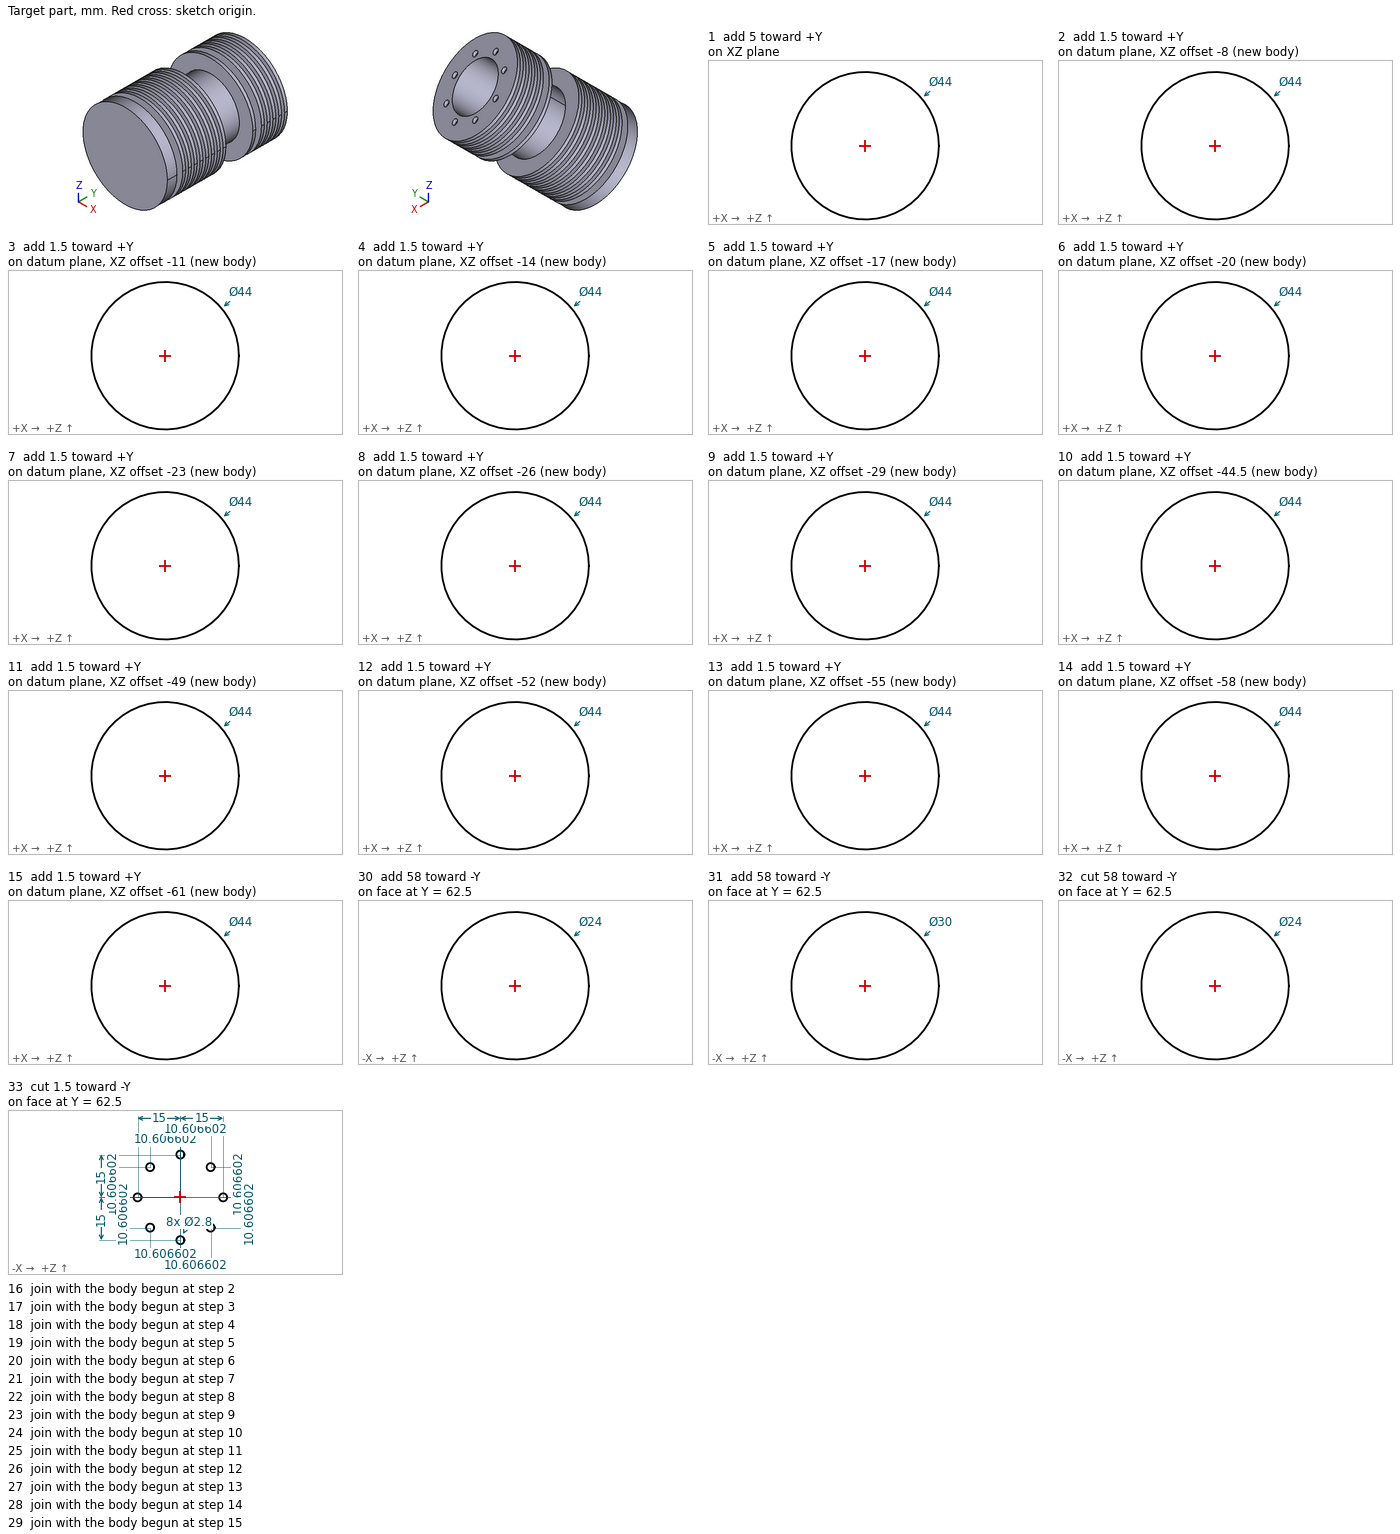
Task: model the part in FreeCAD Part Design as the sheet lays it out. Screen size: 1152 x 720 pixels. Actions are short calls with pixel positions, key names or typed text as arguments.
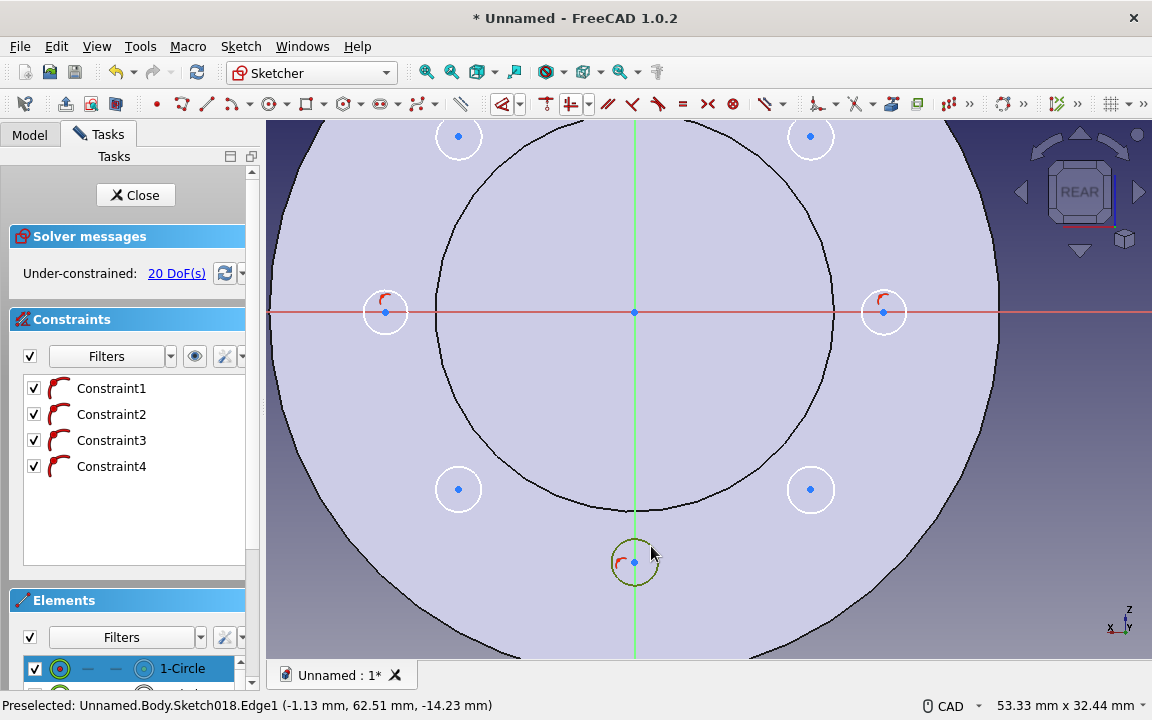
click(475, 473)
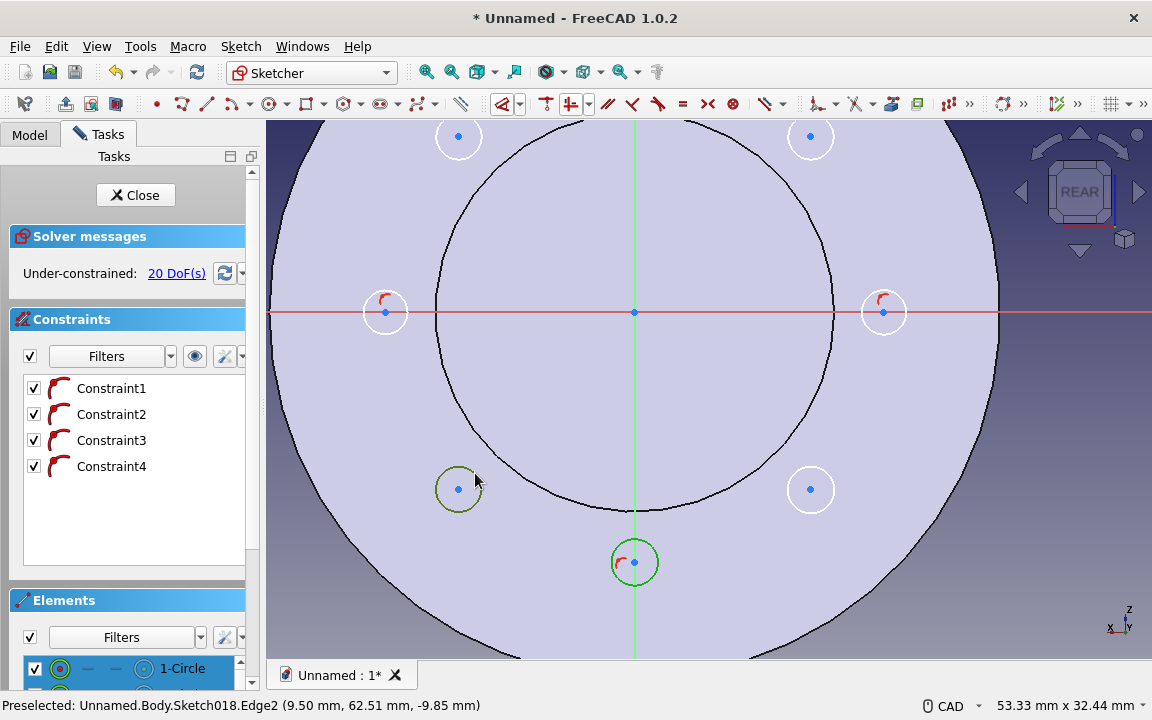
click(401, 297)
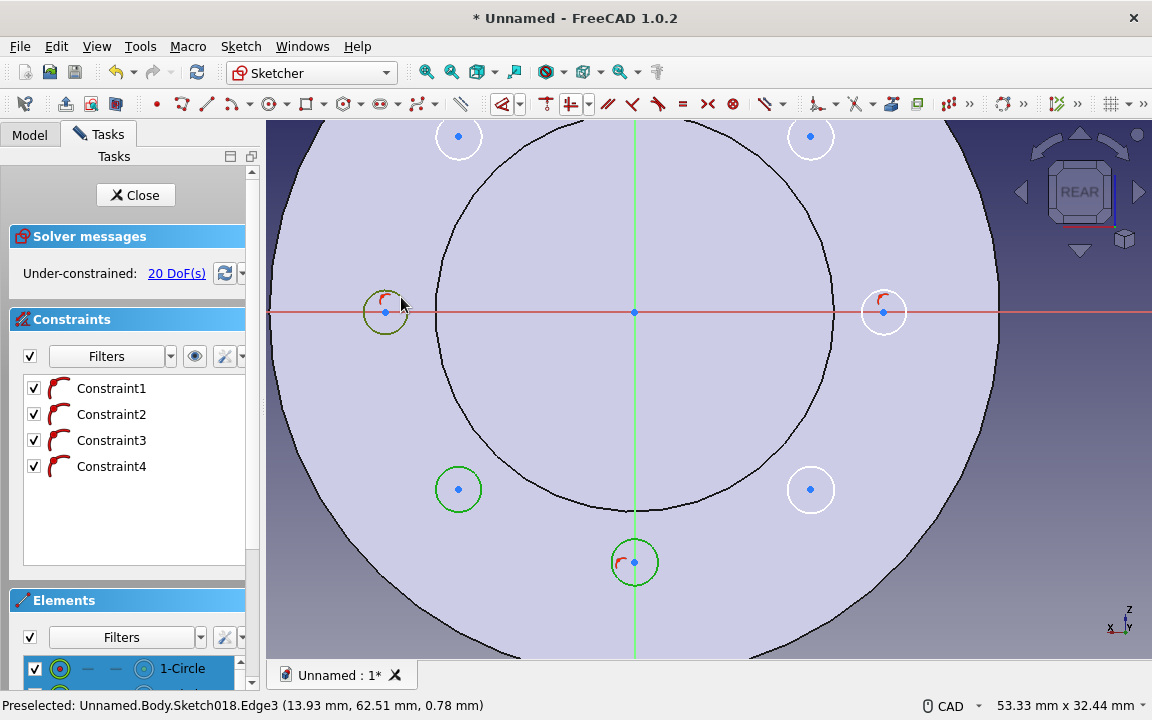
click(443, 153)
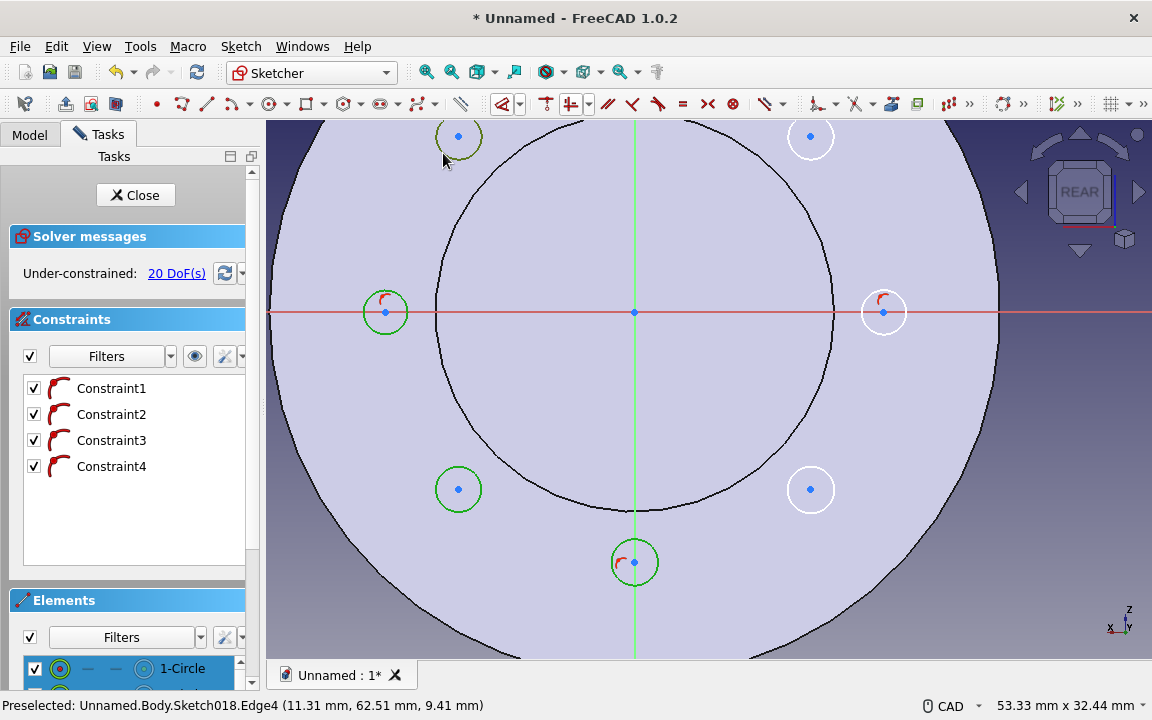
scroll(652, 546, down, 2)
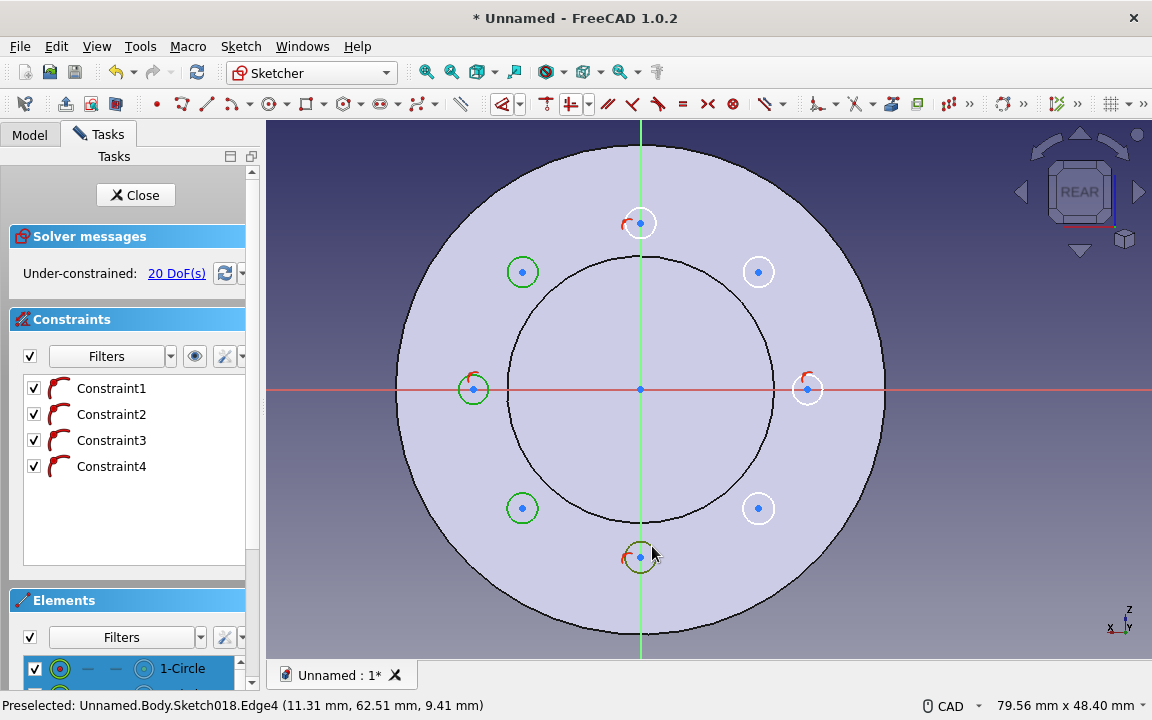
scroll(651, 212, up, 2)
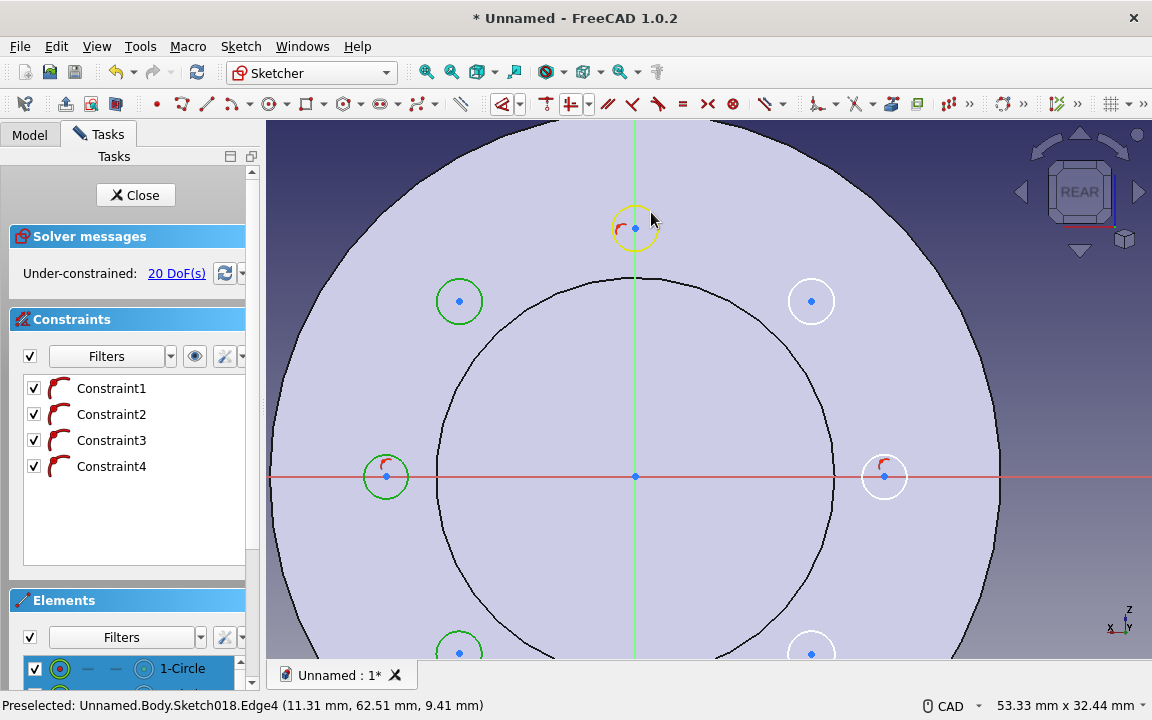
click(651, 212)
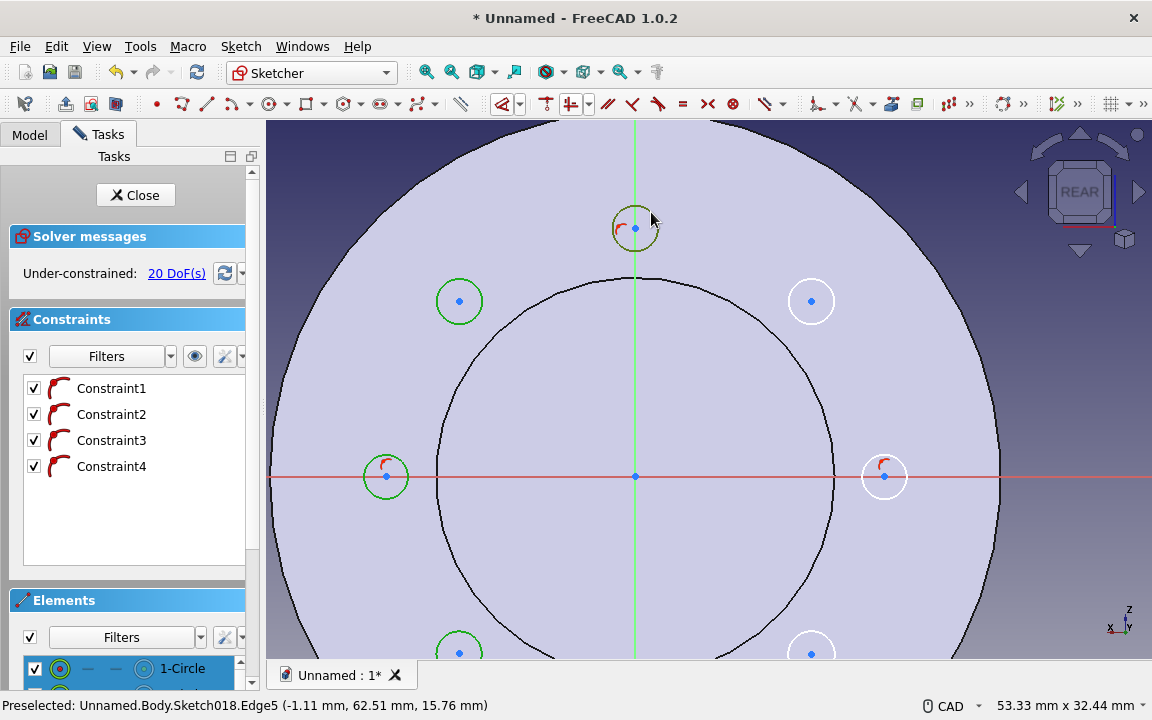
click(827, 286)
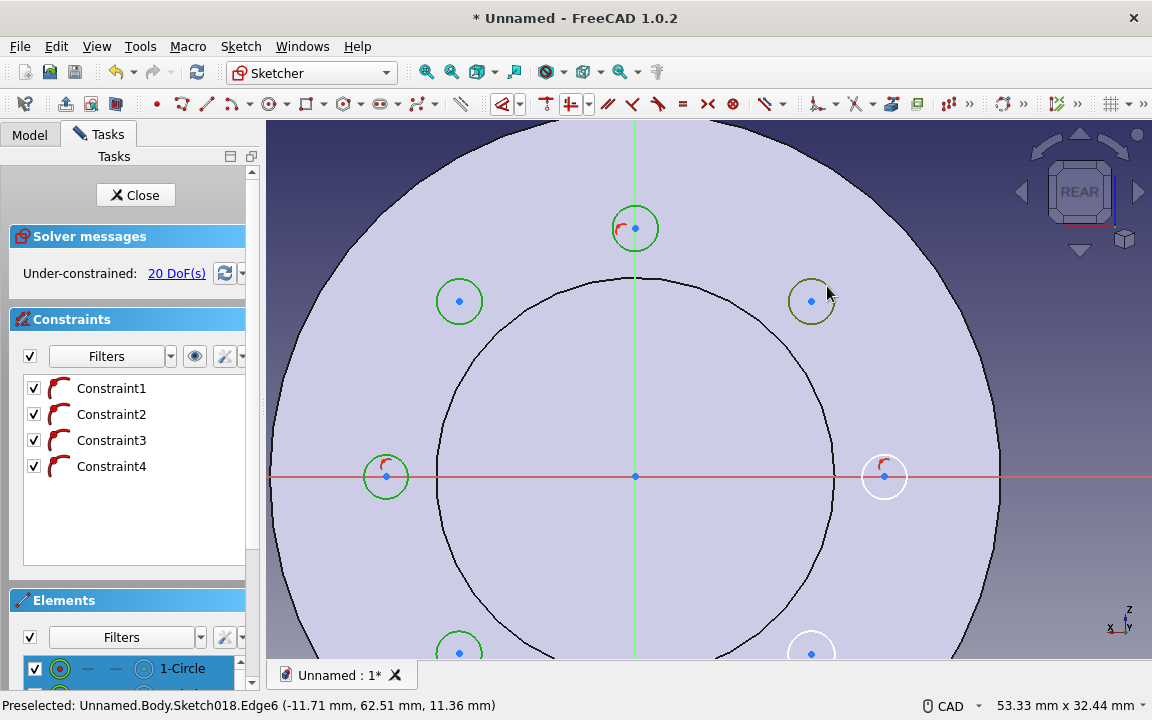
click(900, 461)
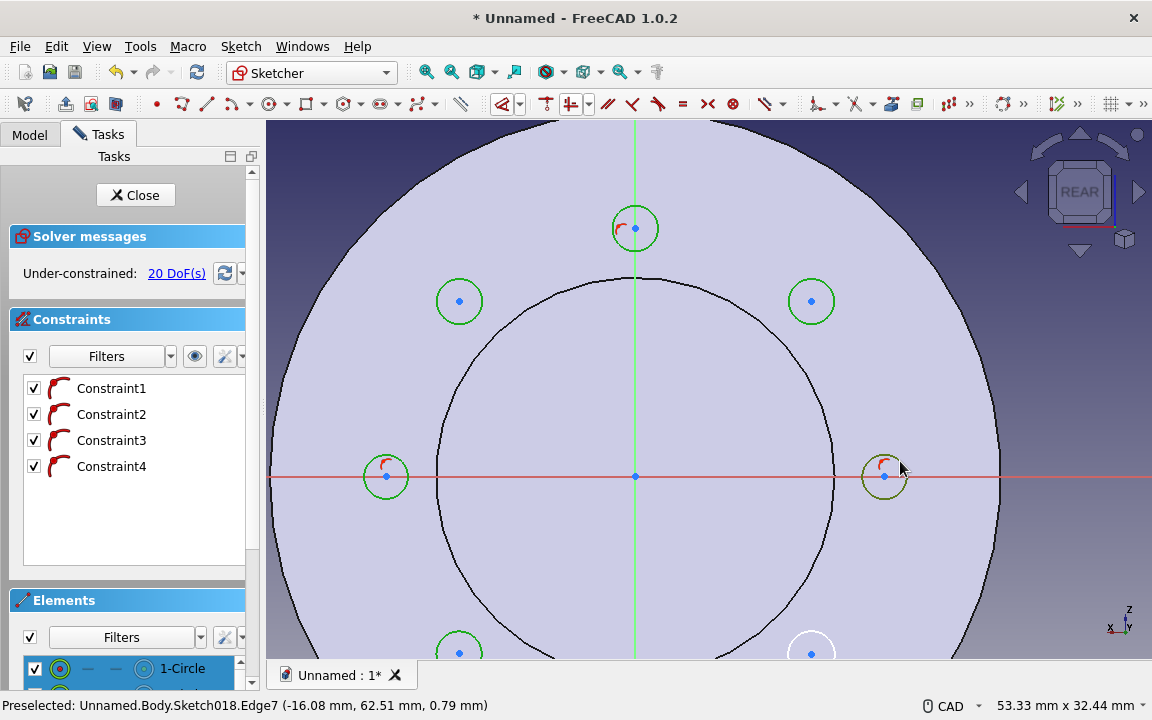
scroll(651, 212, down, 2)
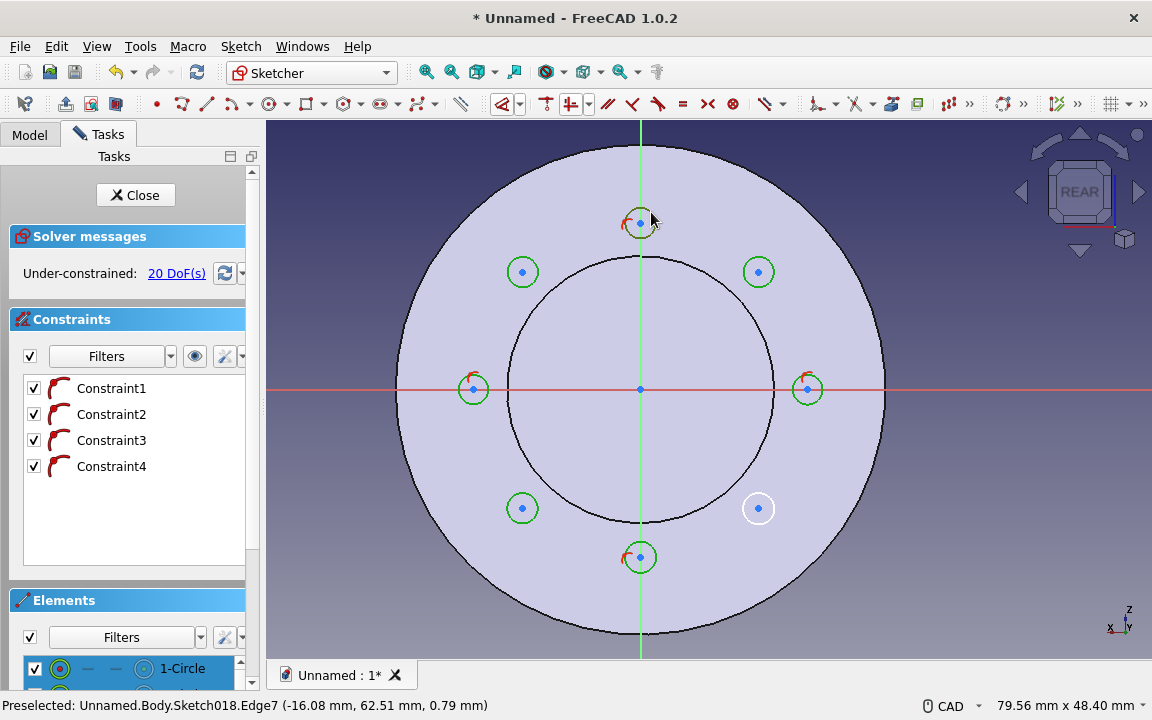
click(770, 498)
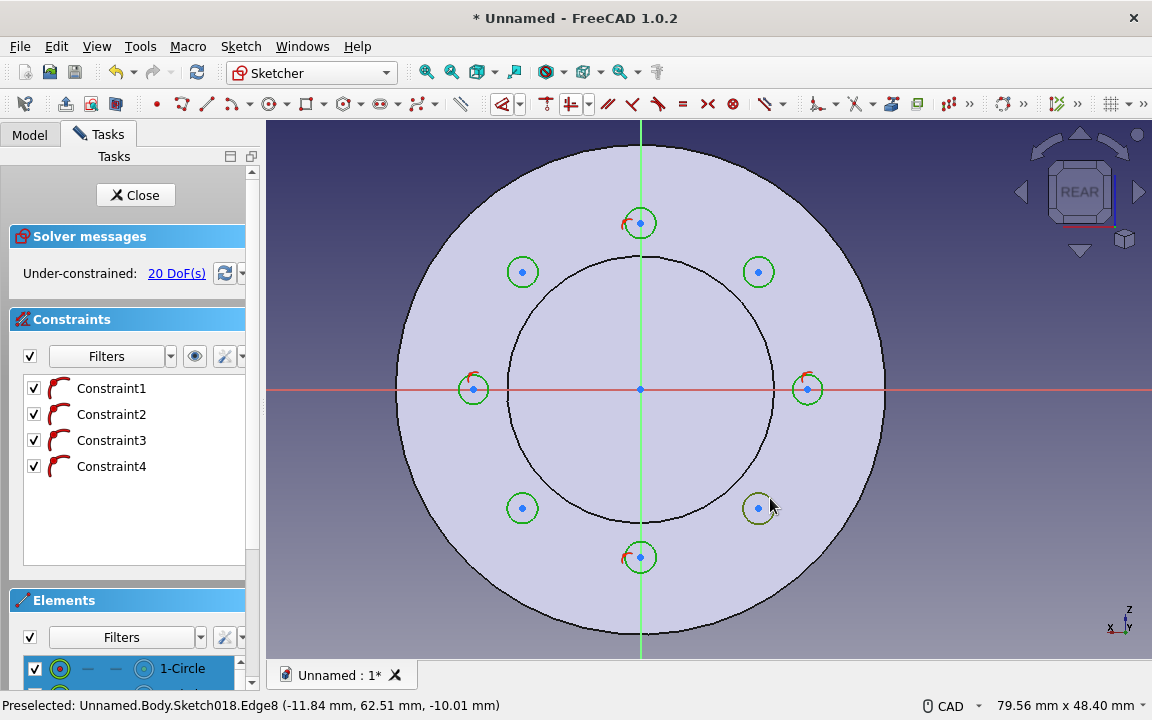
key(e)